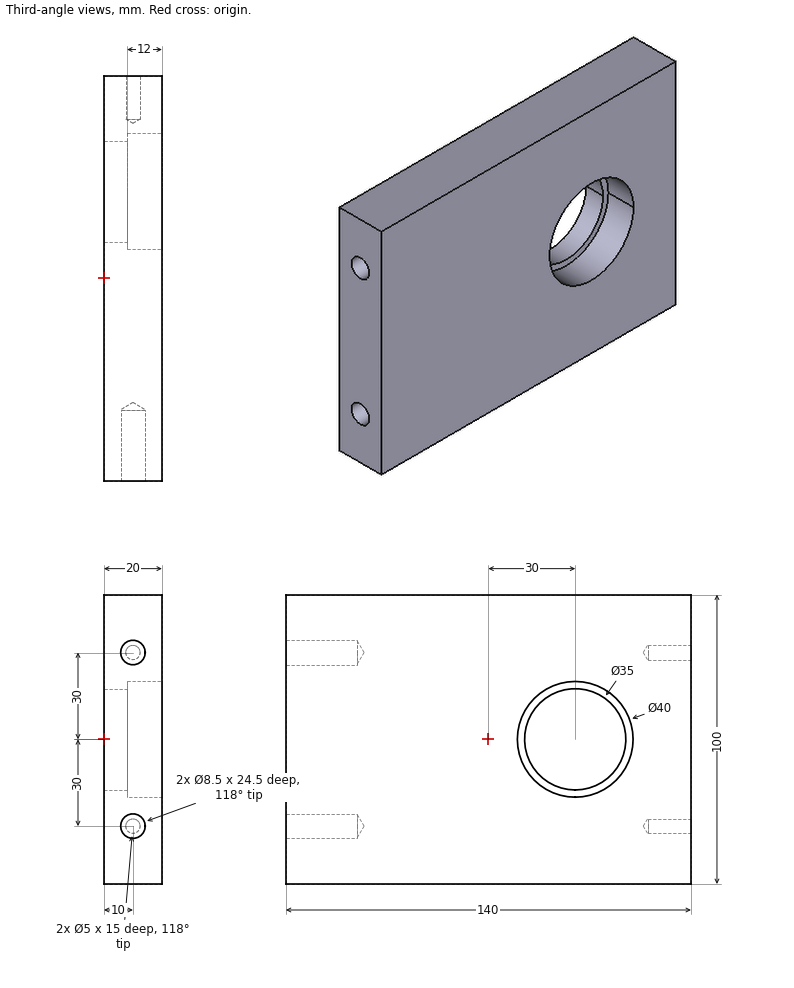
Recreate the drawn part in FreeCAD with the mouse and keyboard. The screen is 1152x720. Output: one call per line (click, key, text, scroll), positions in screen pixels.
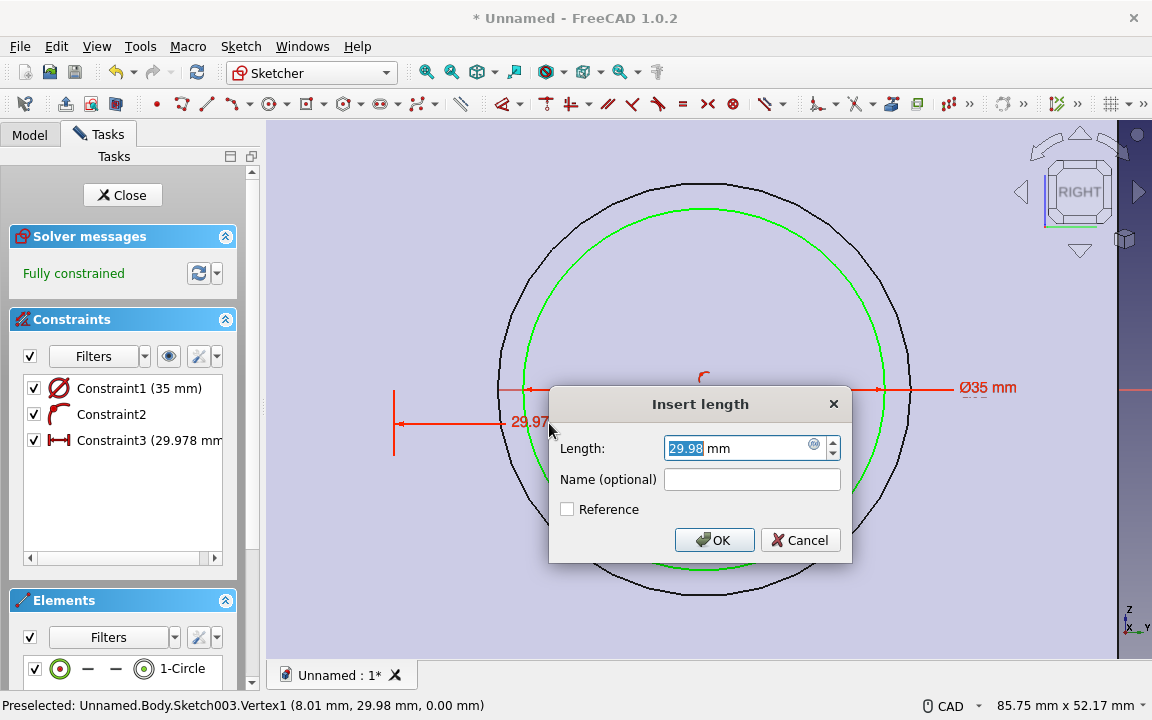
text(30)
key(Return)
key(Escape)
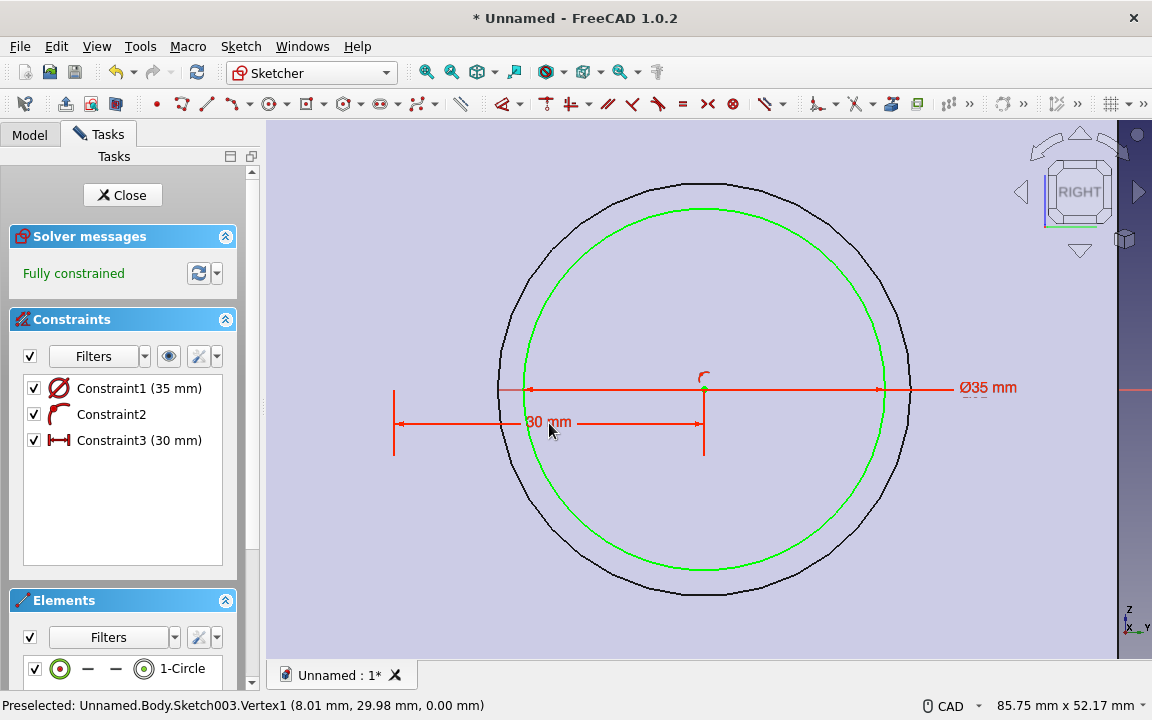
click(123, 195)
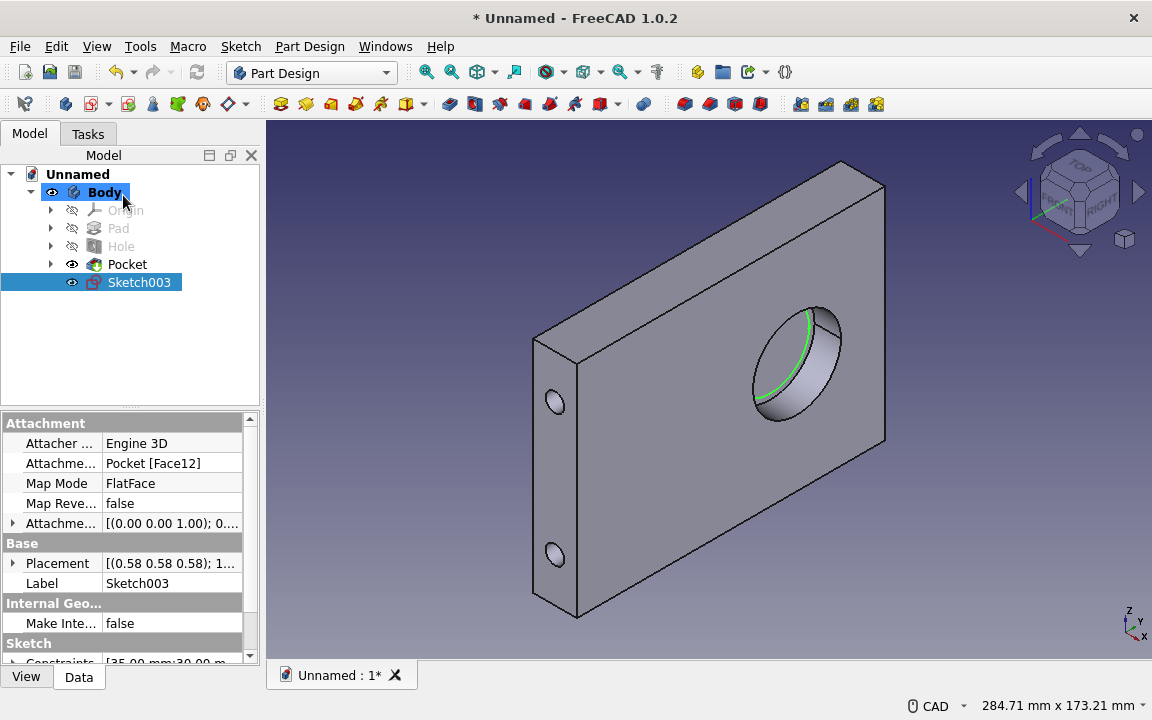
click(450, 104)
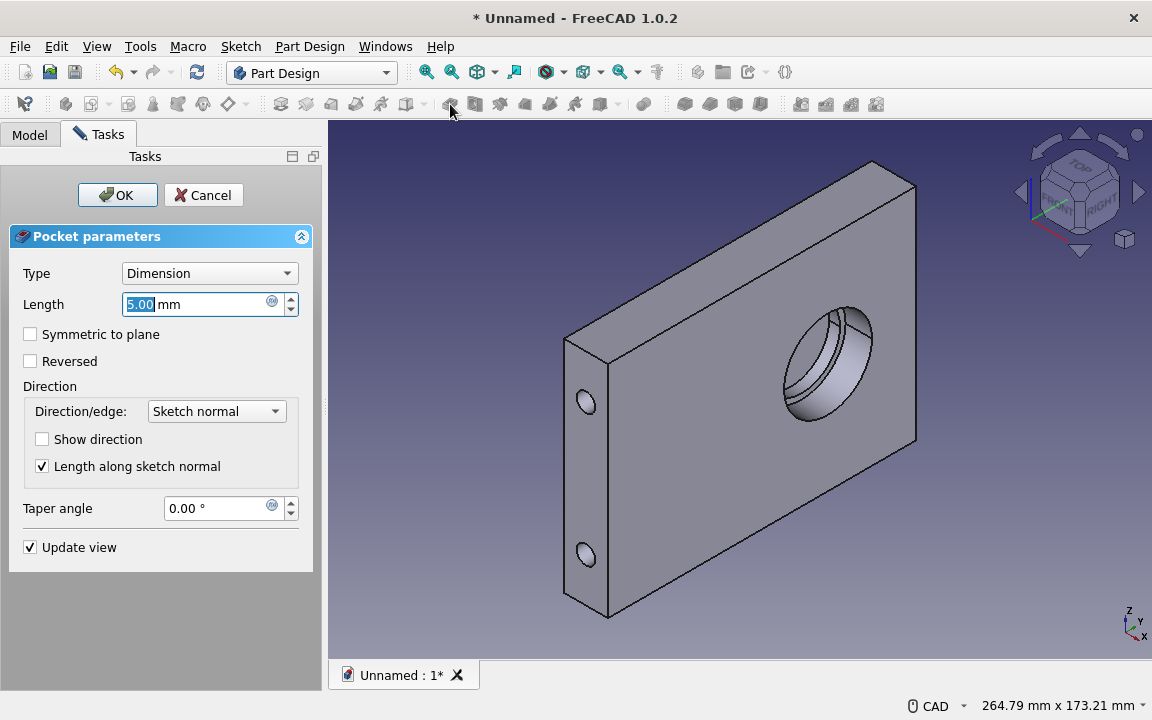
click(210, 274)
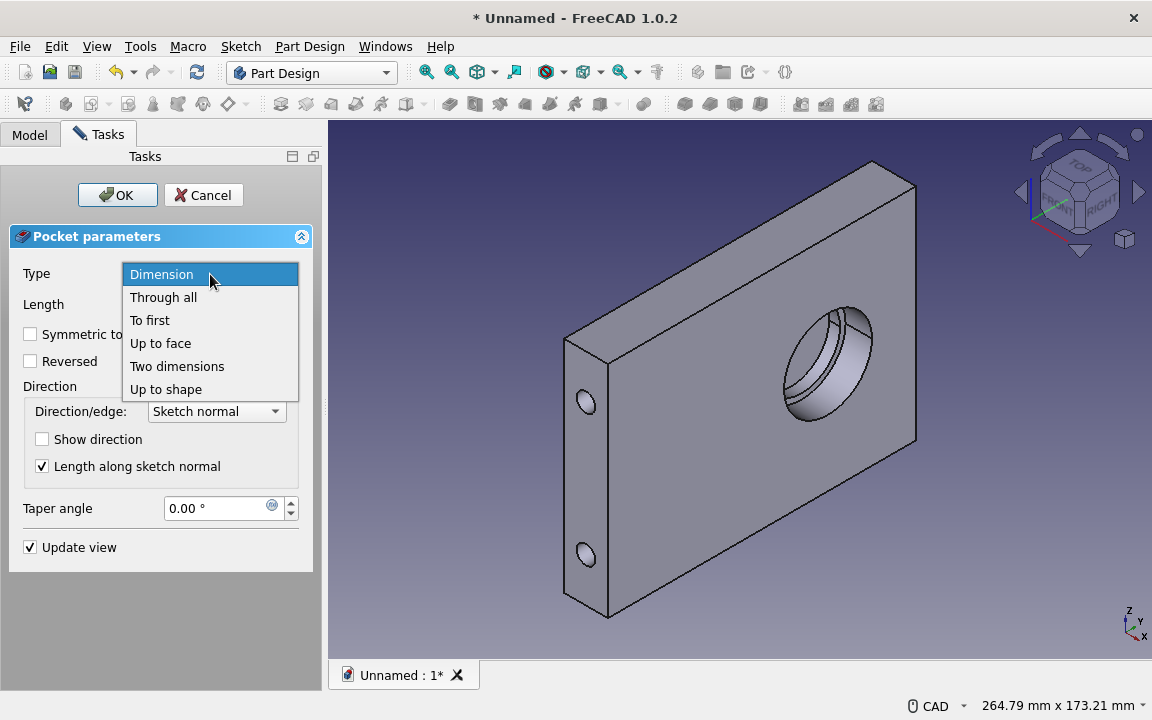
click(208, 298)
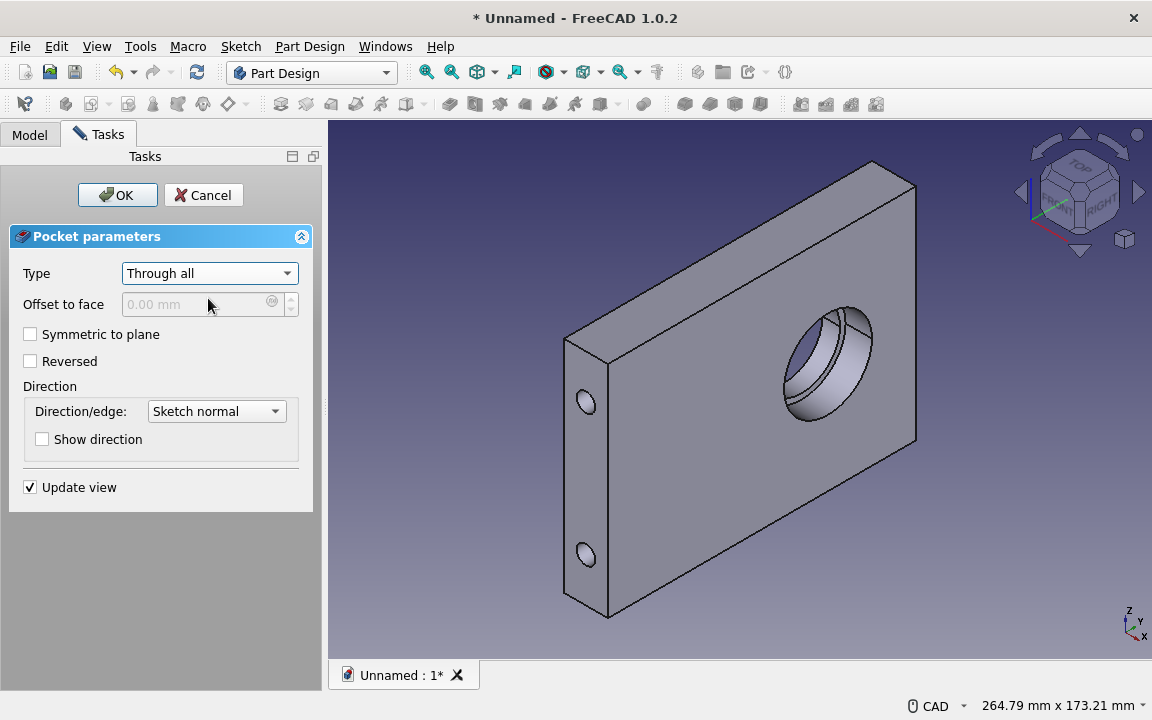
click(118, 195)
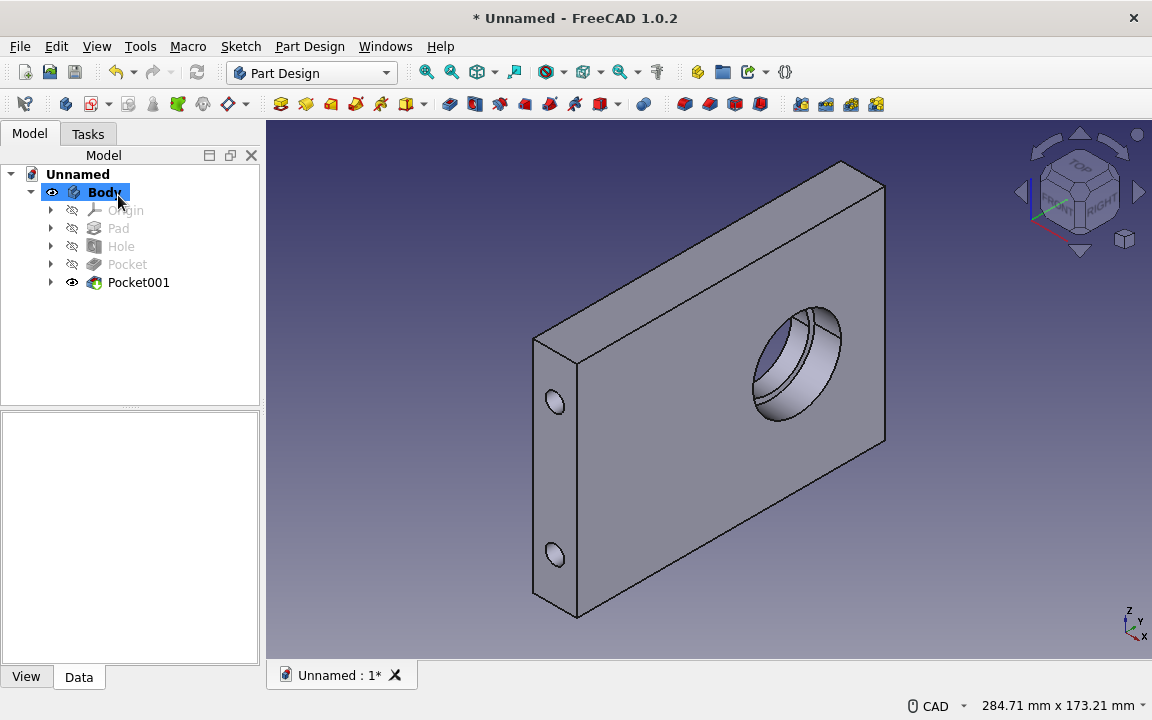
key(4)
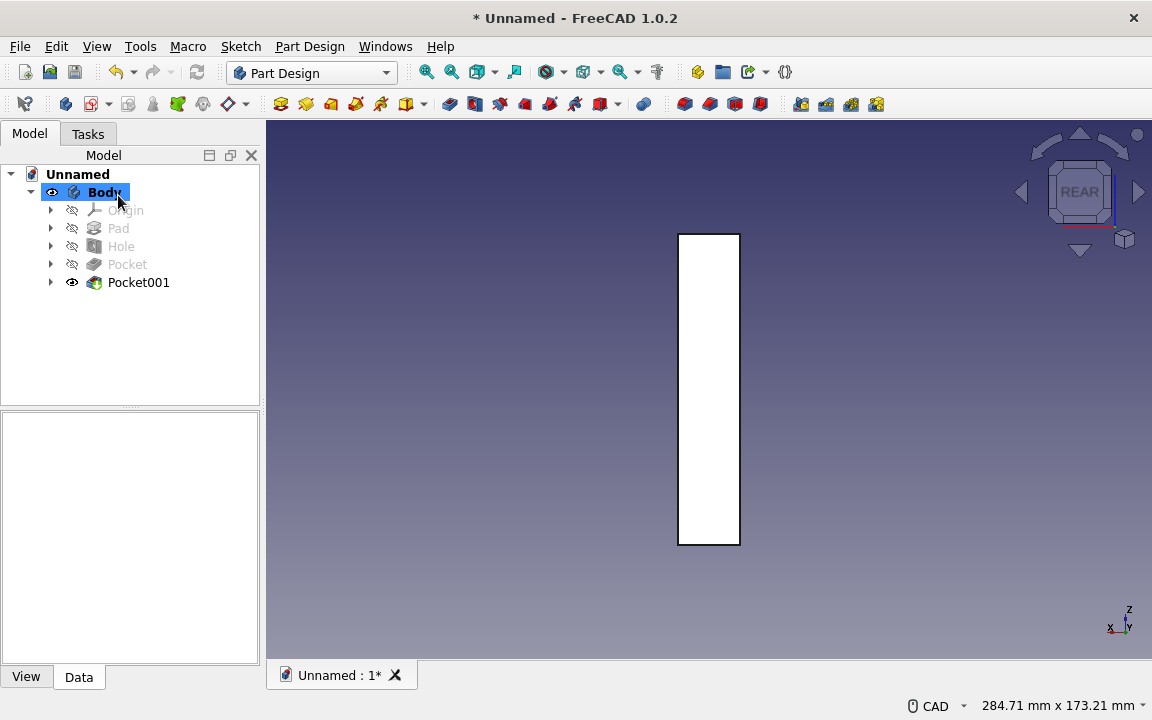
click(709, 477)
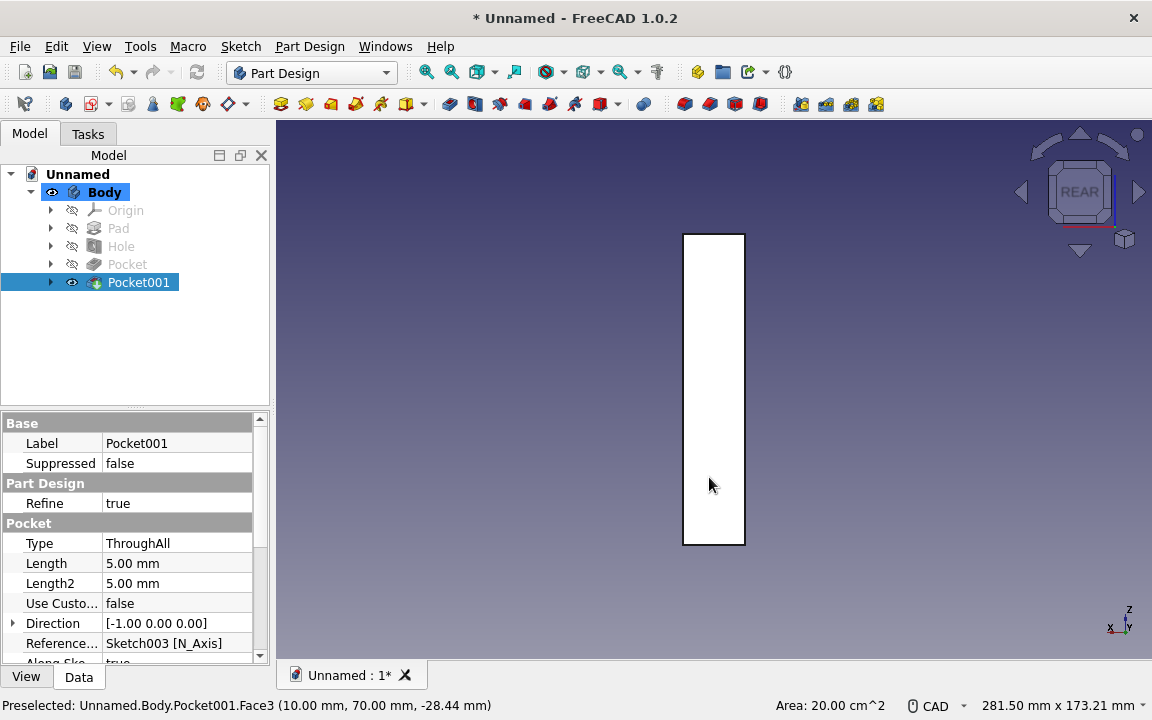
click(90, 104)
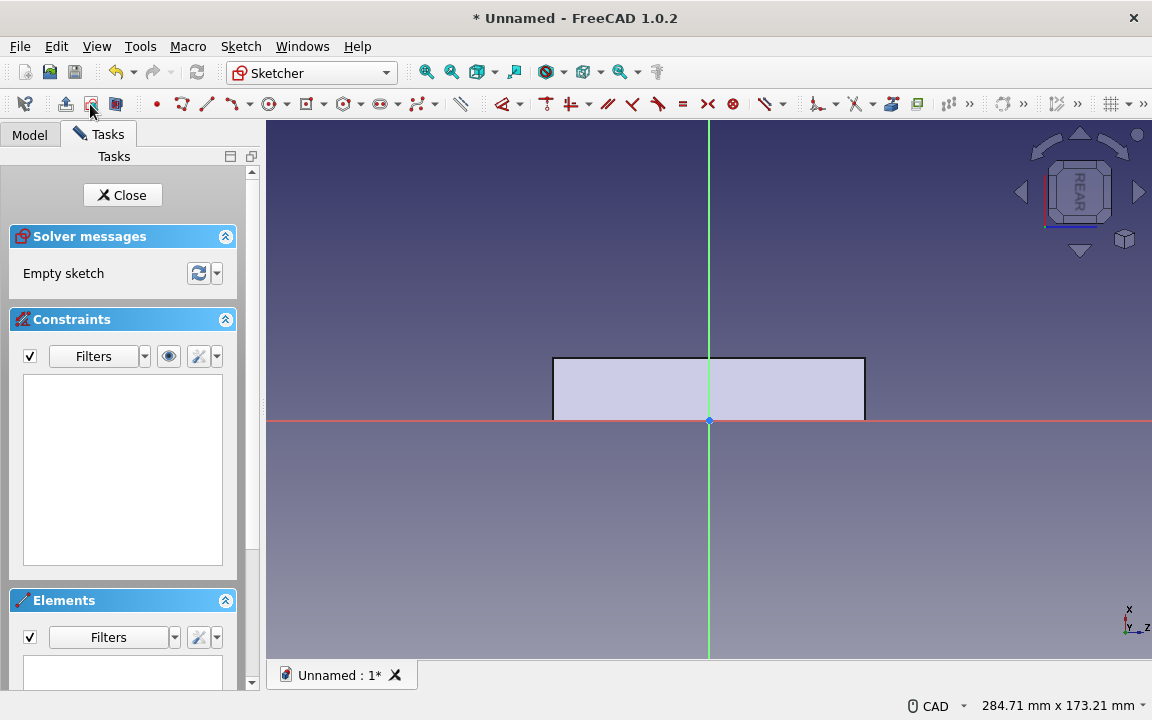
scroll(765, 411, up, 4)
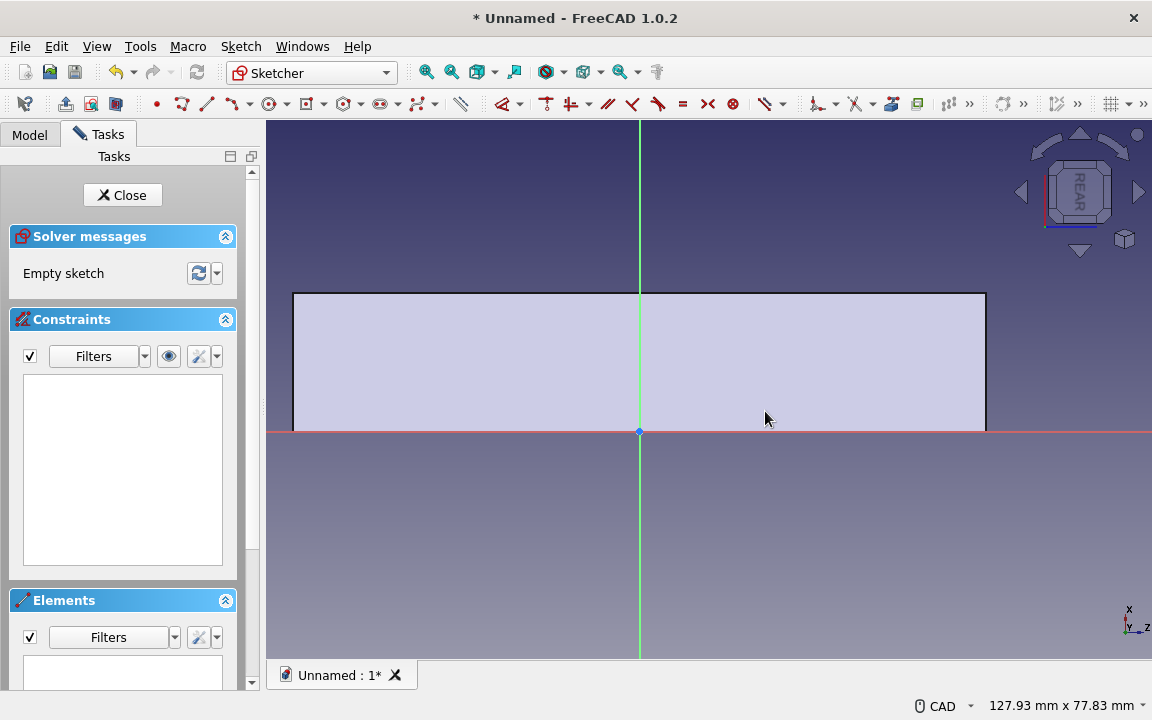
key(g)
key(c)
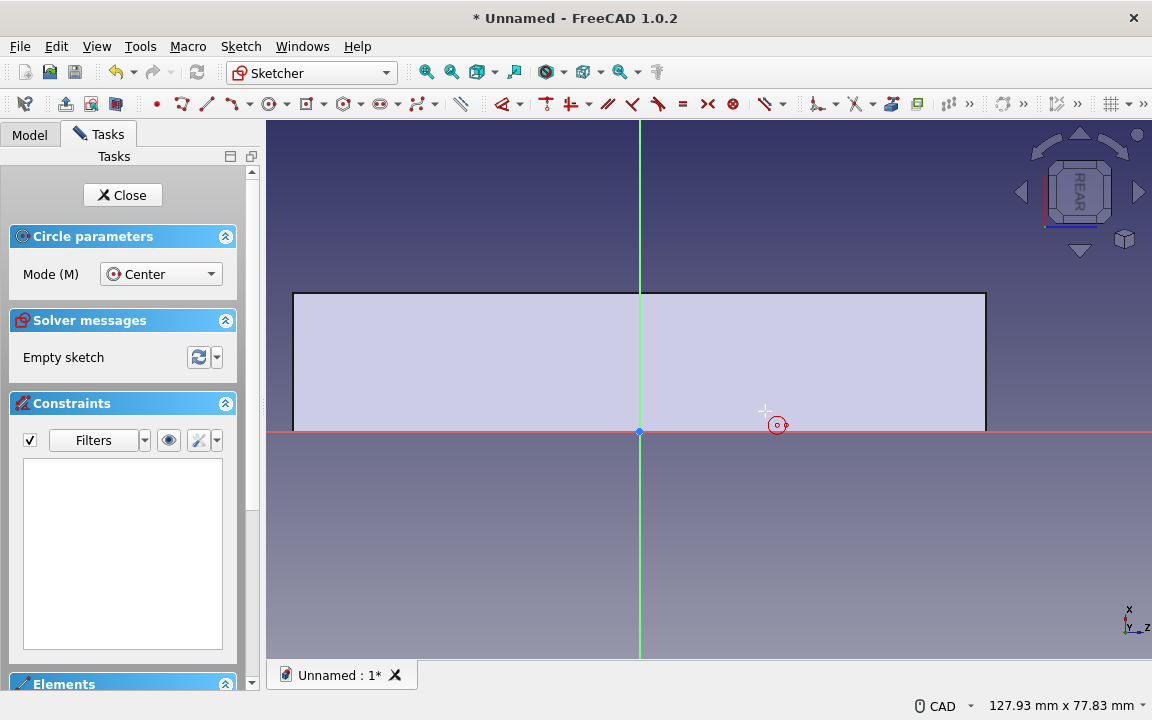
scroll(432, 362, up, 2)